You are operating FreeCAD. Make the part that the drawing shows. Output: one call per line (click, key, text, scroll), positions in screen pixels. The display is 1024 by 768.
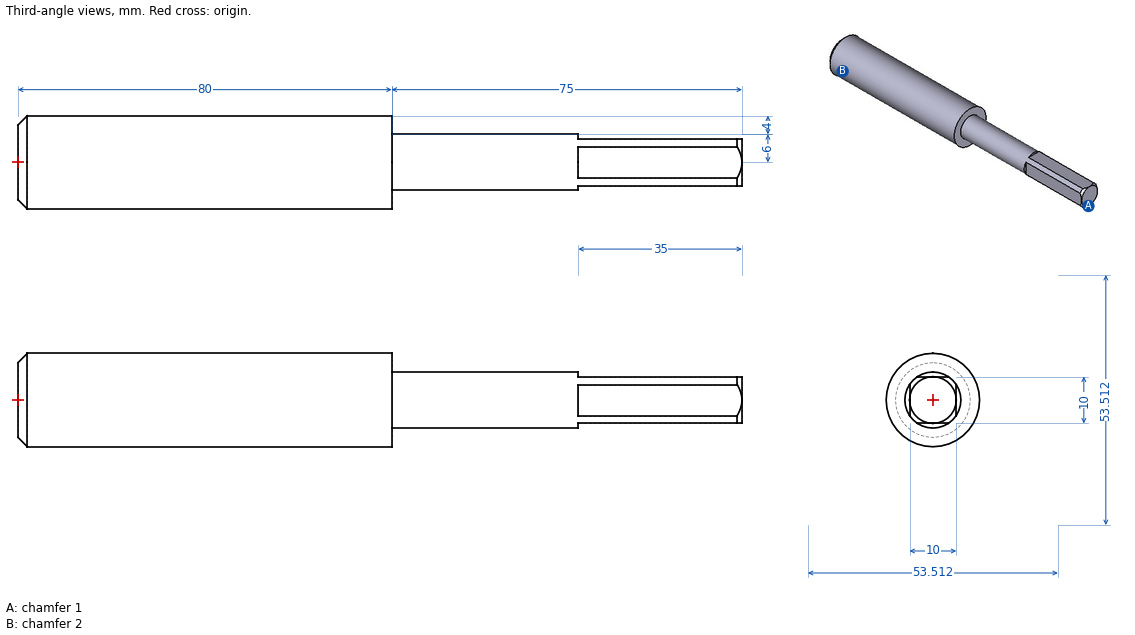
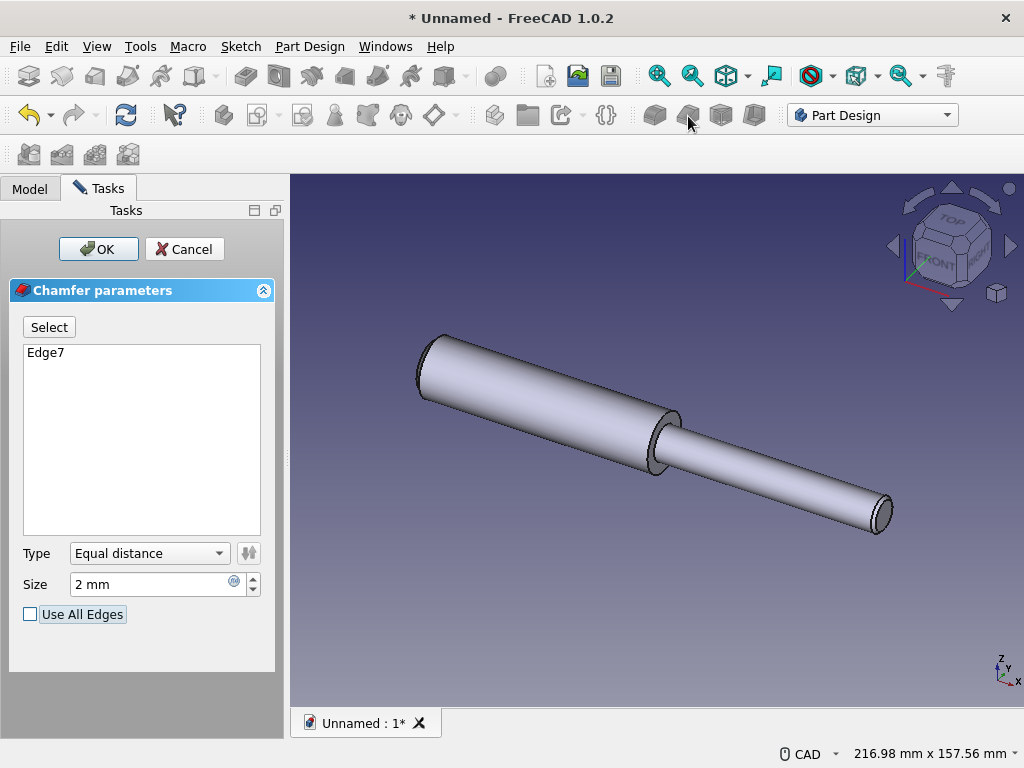
click(99, 249)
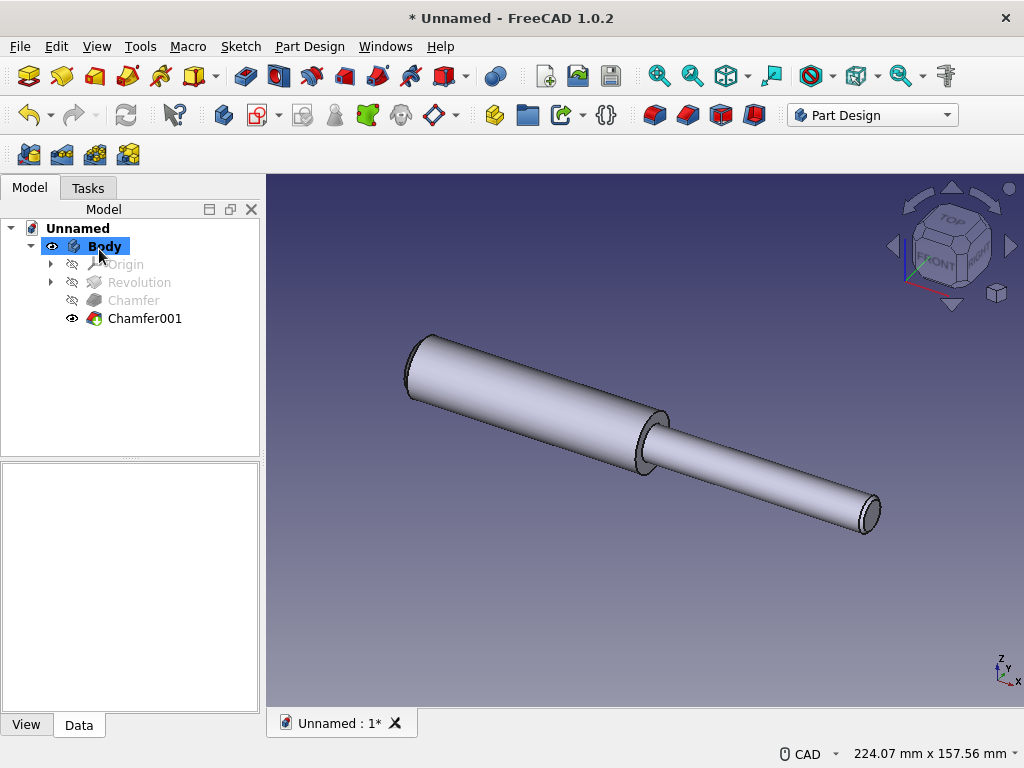
click(874, 516)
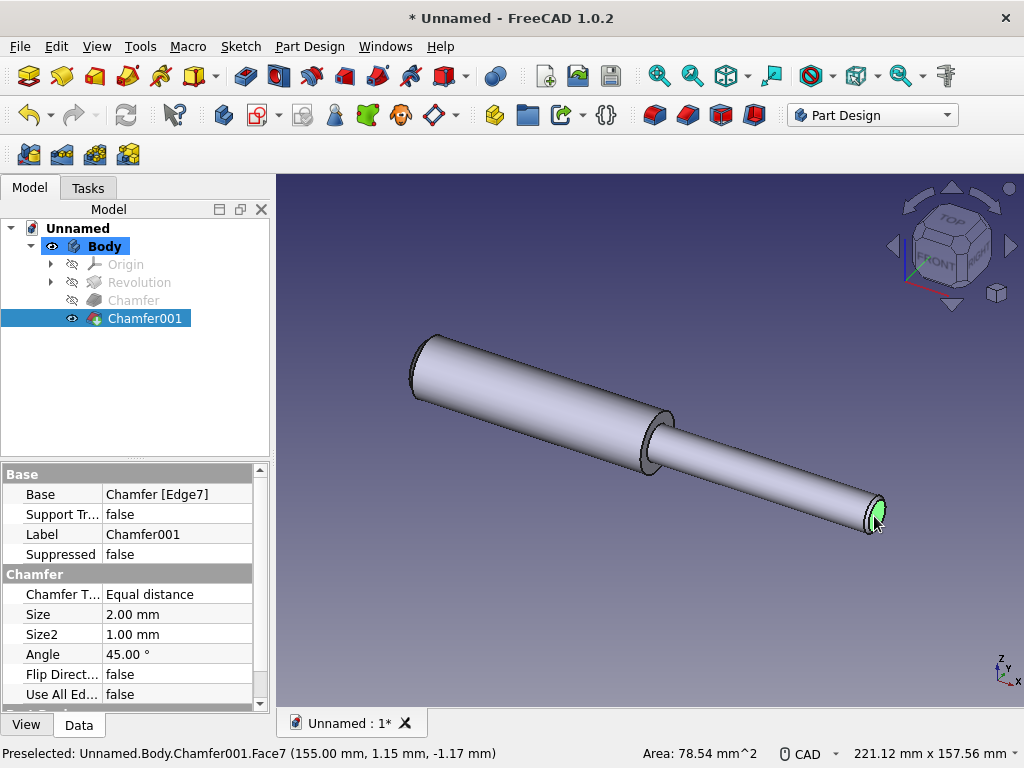
click(256, 116)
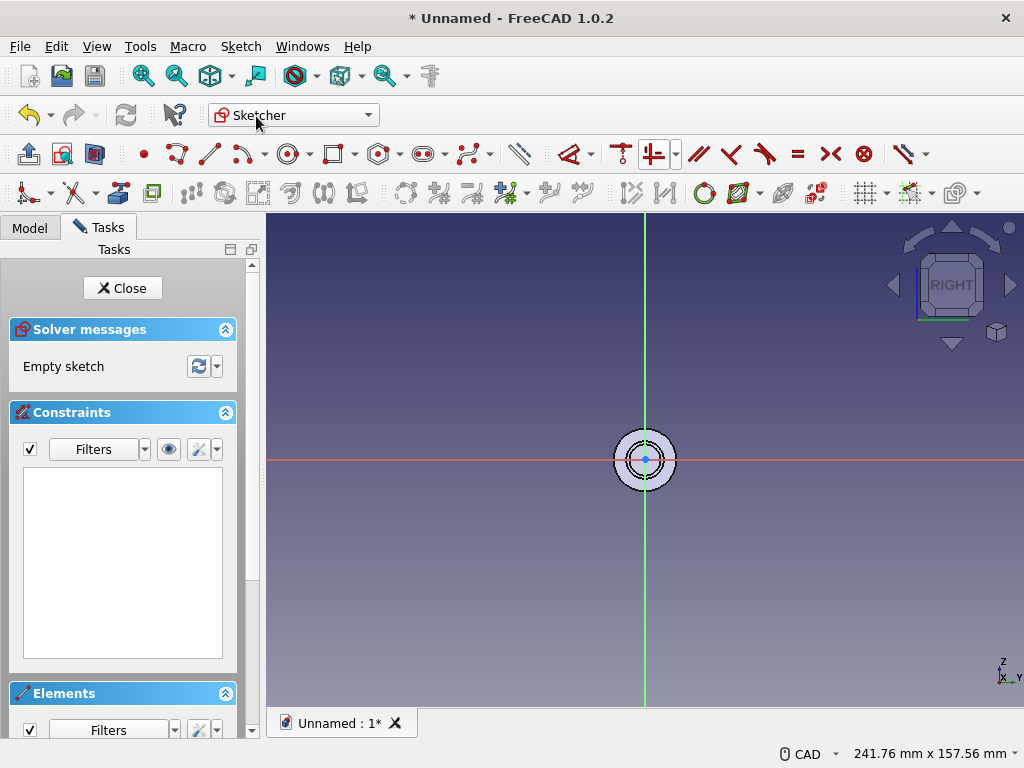
scroll(728, 460, up, 3)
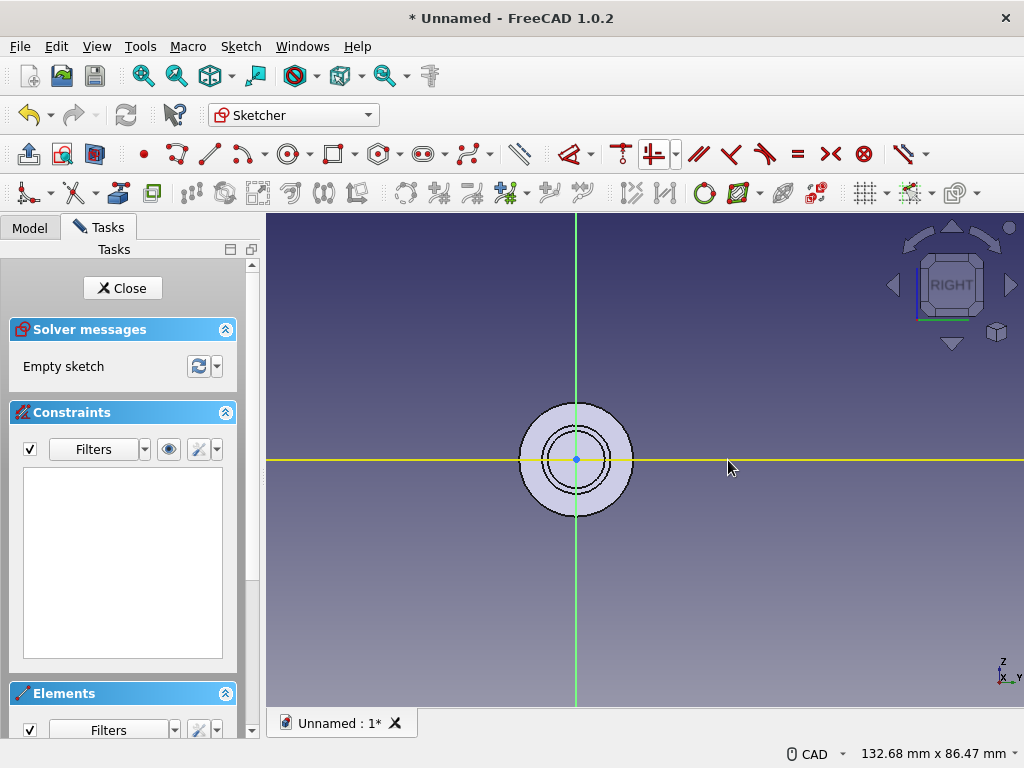
key(g)
key(v)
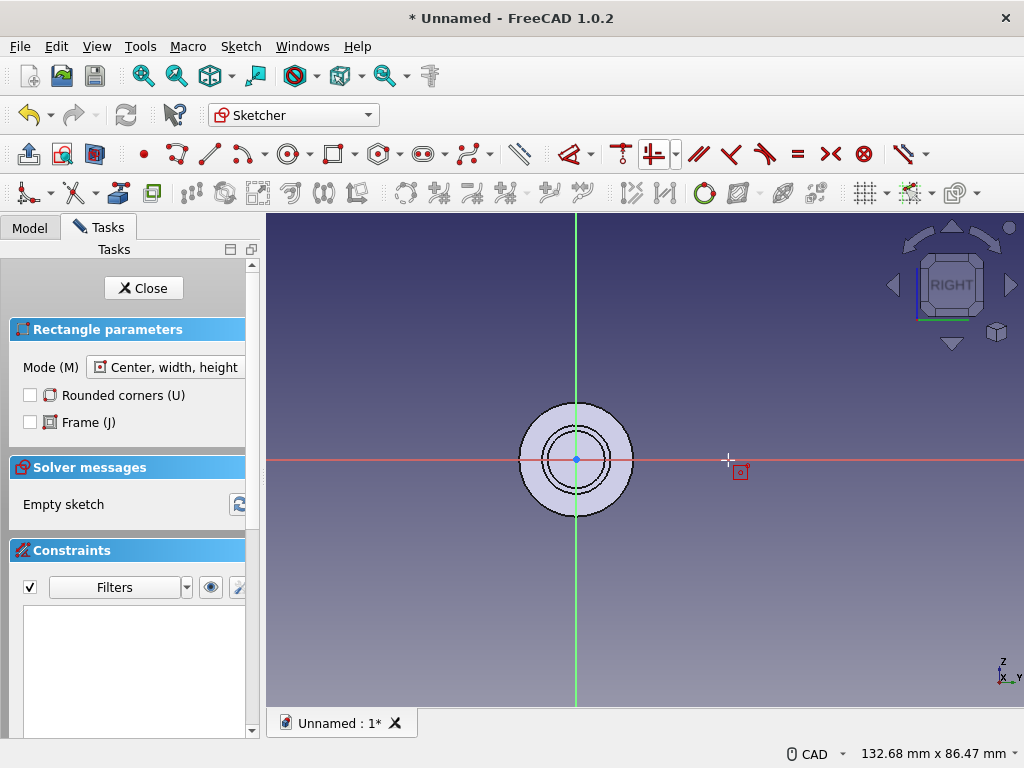
click(576, 460)
click(729, 307)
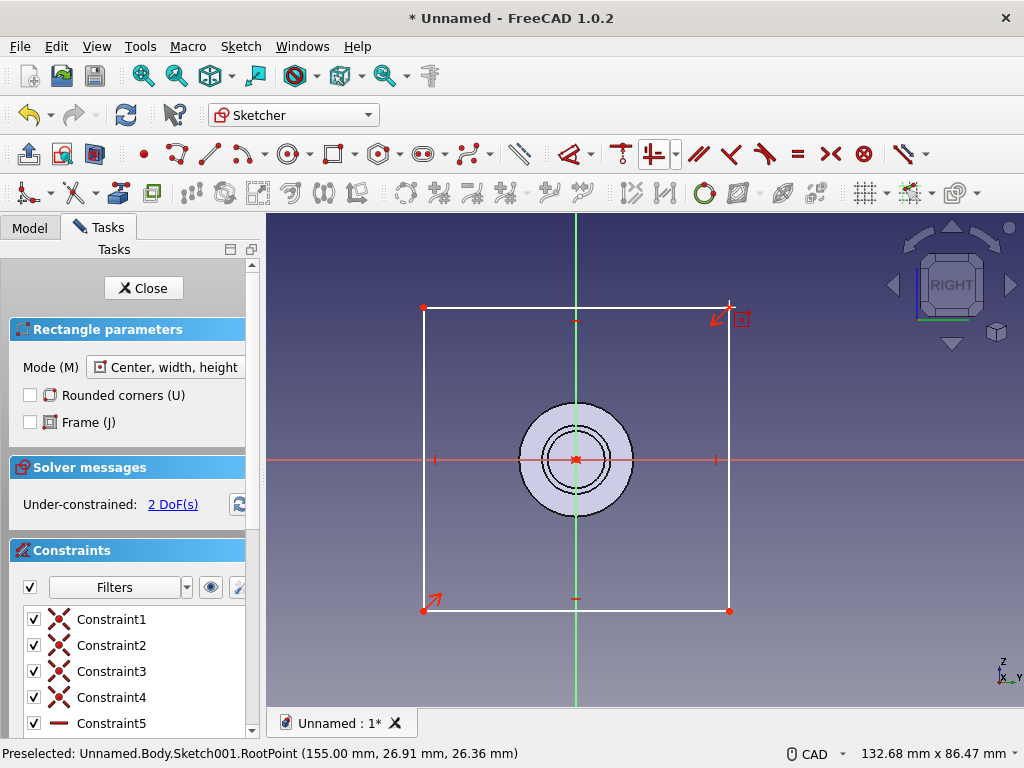
click(576, 460)
click(605, 431)
key(Escape)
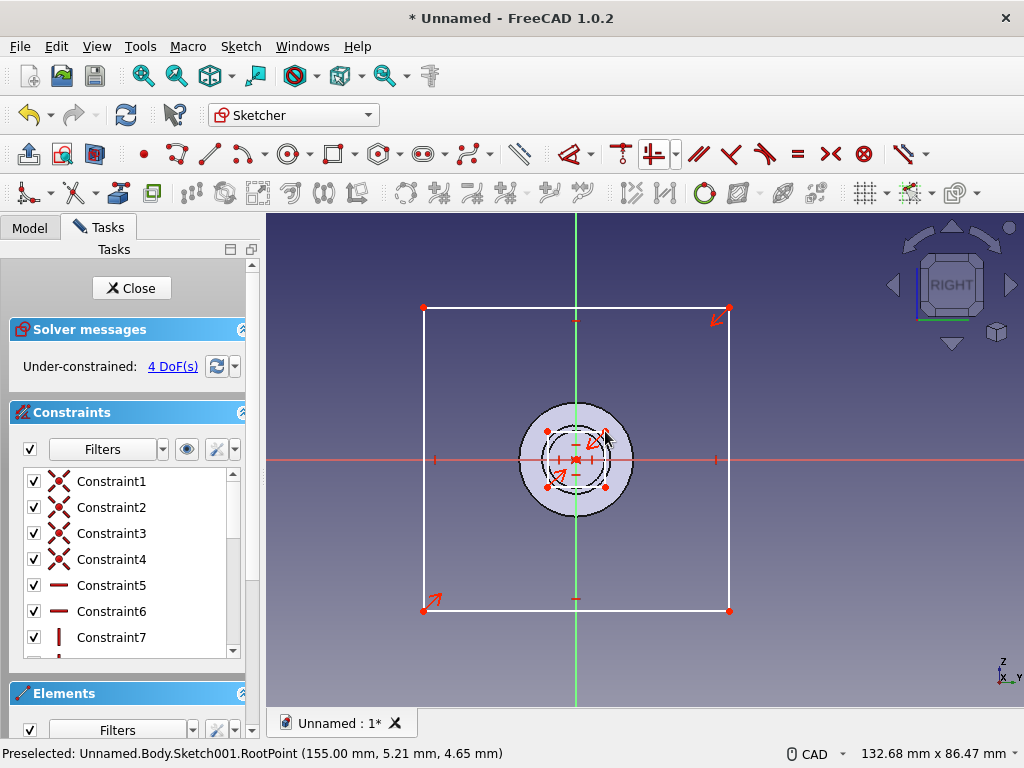
click(568, 154)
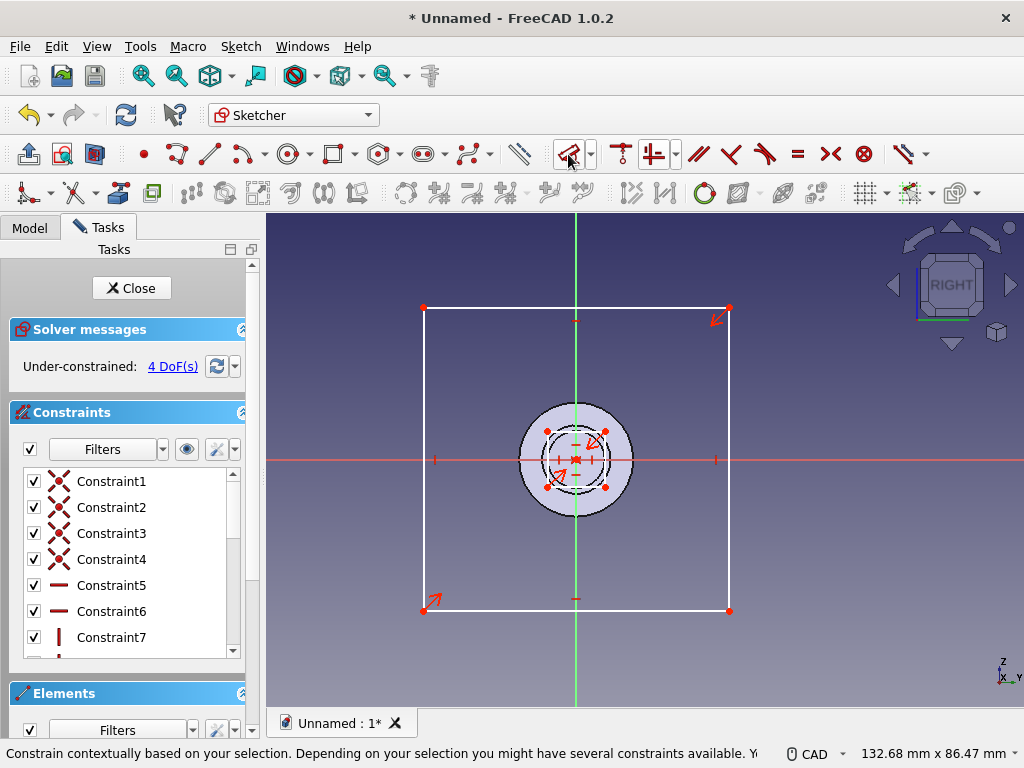
click(565, 487)
click(563, 521)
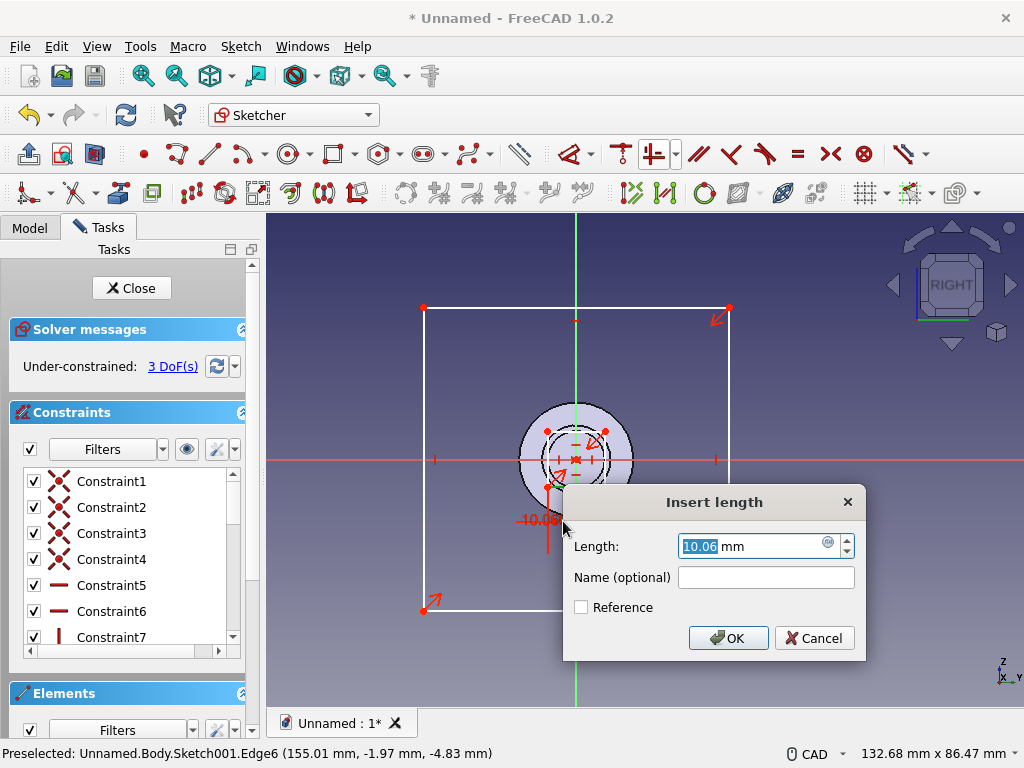
text(10)
key(Return)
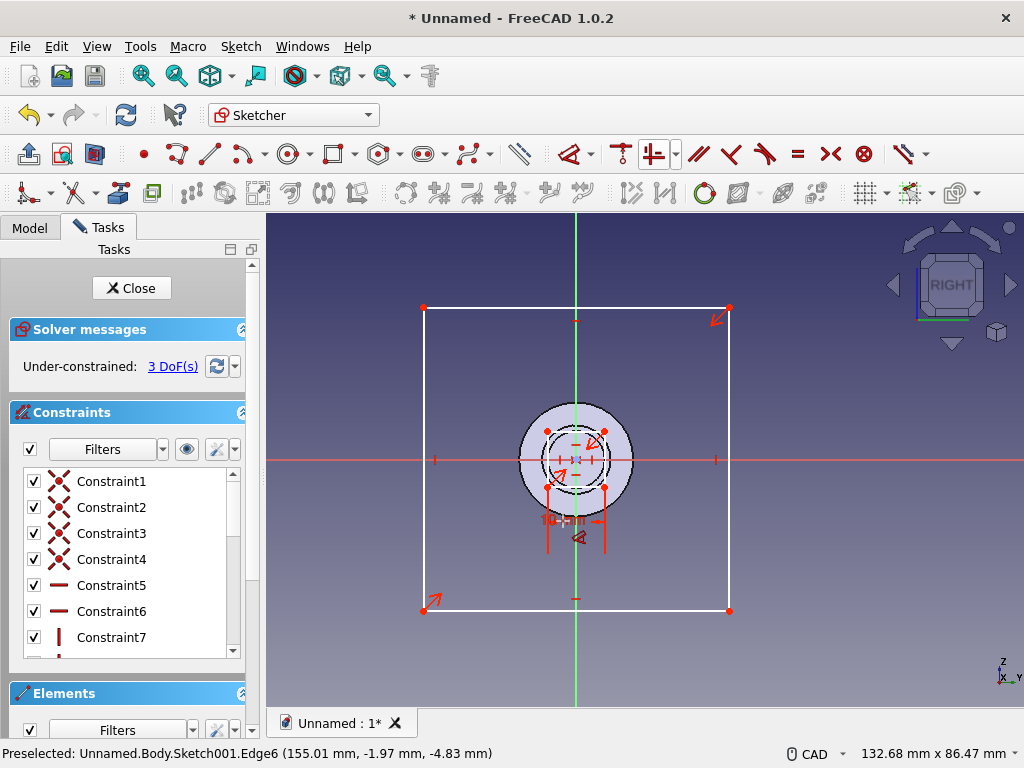
scroll(605, 471, up, 2)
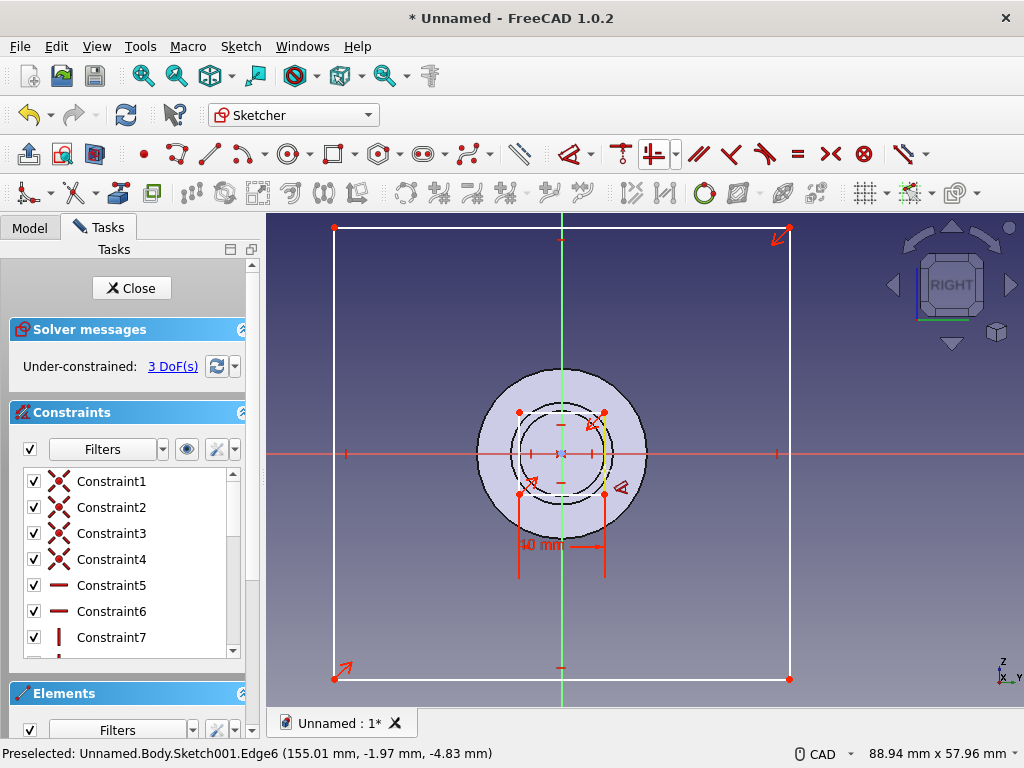
click(605, 470)
click(639, 435)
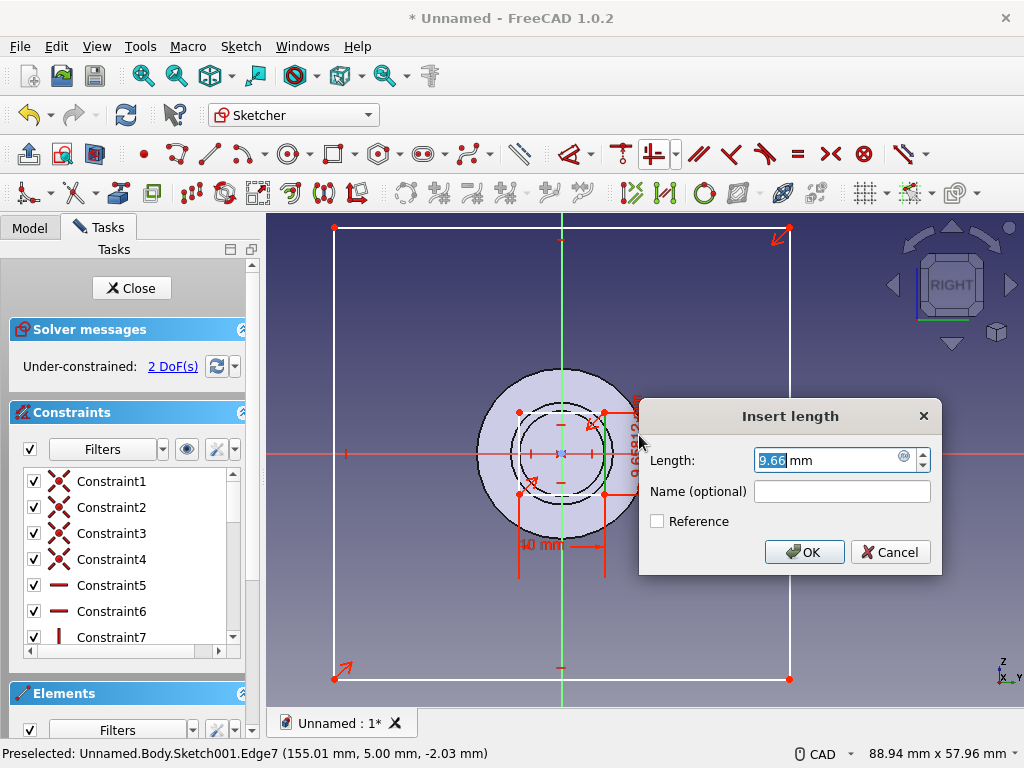
text(10)
key(Return)